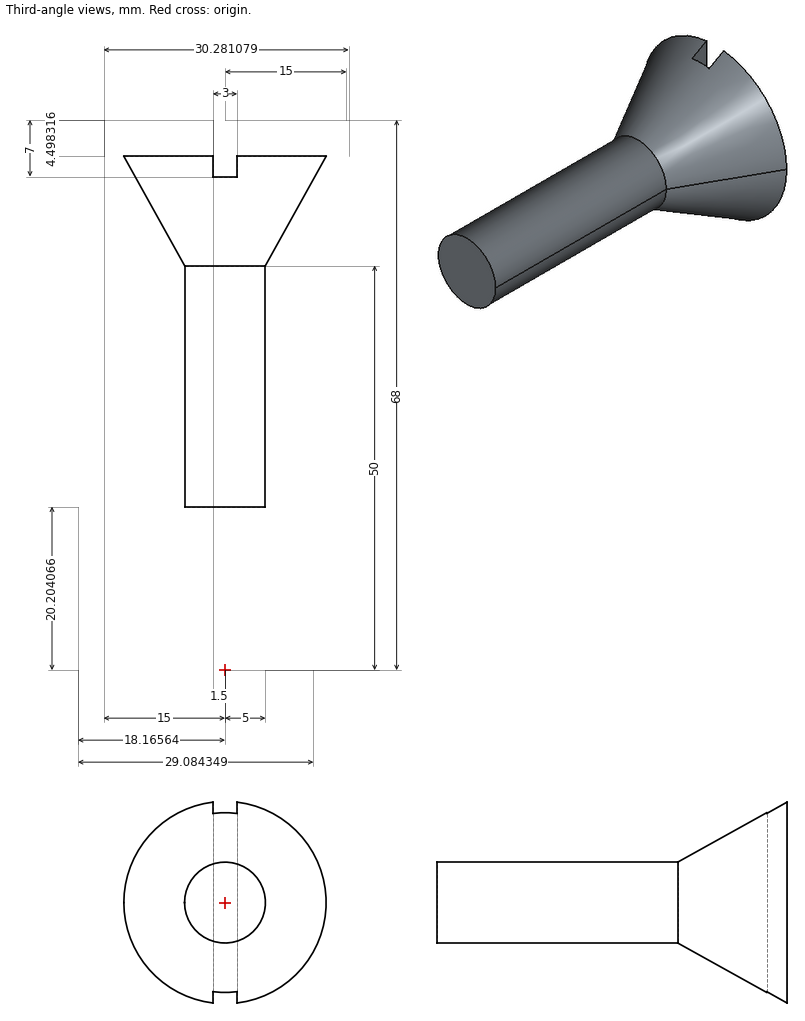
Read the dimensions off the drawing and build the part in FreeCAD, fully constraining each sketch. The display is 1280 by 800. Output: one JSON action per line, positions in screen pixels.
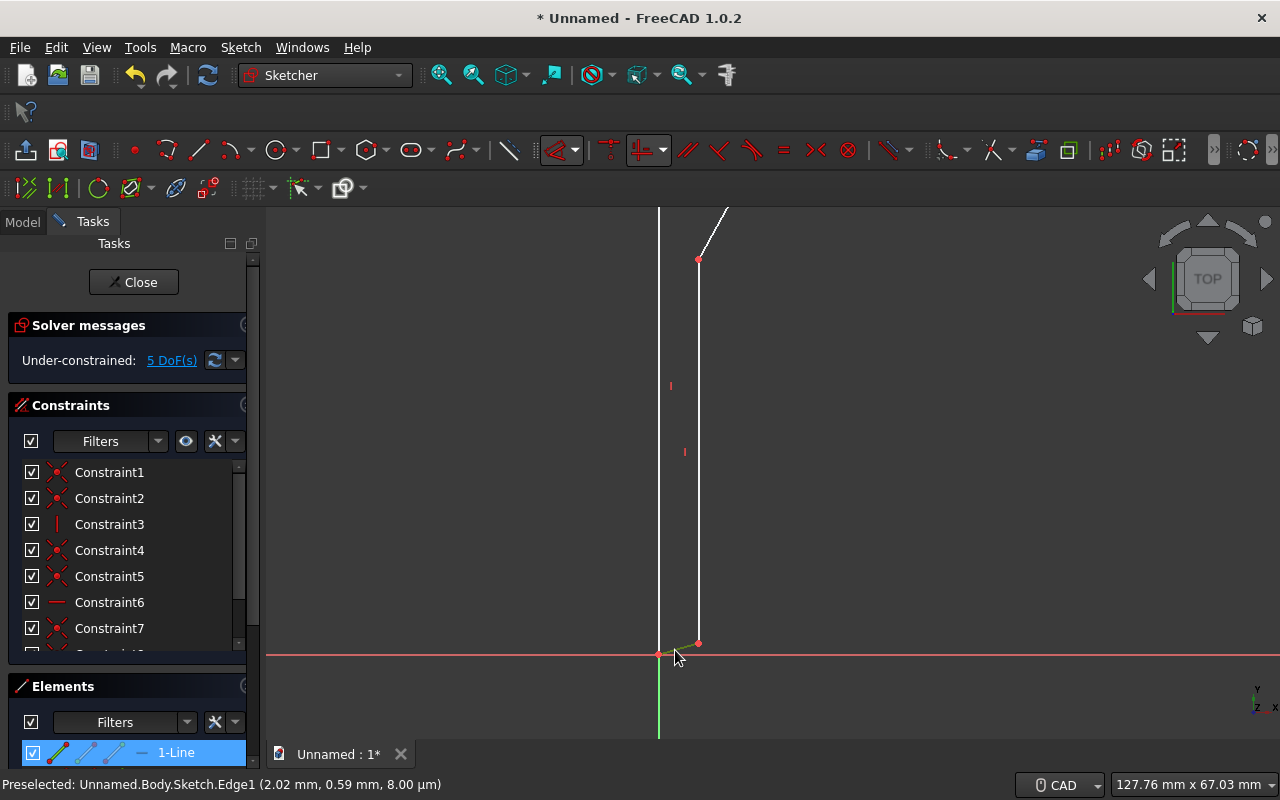
{"action": "left_click", "coordinate": [666, 150]}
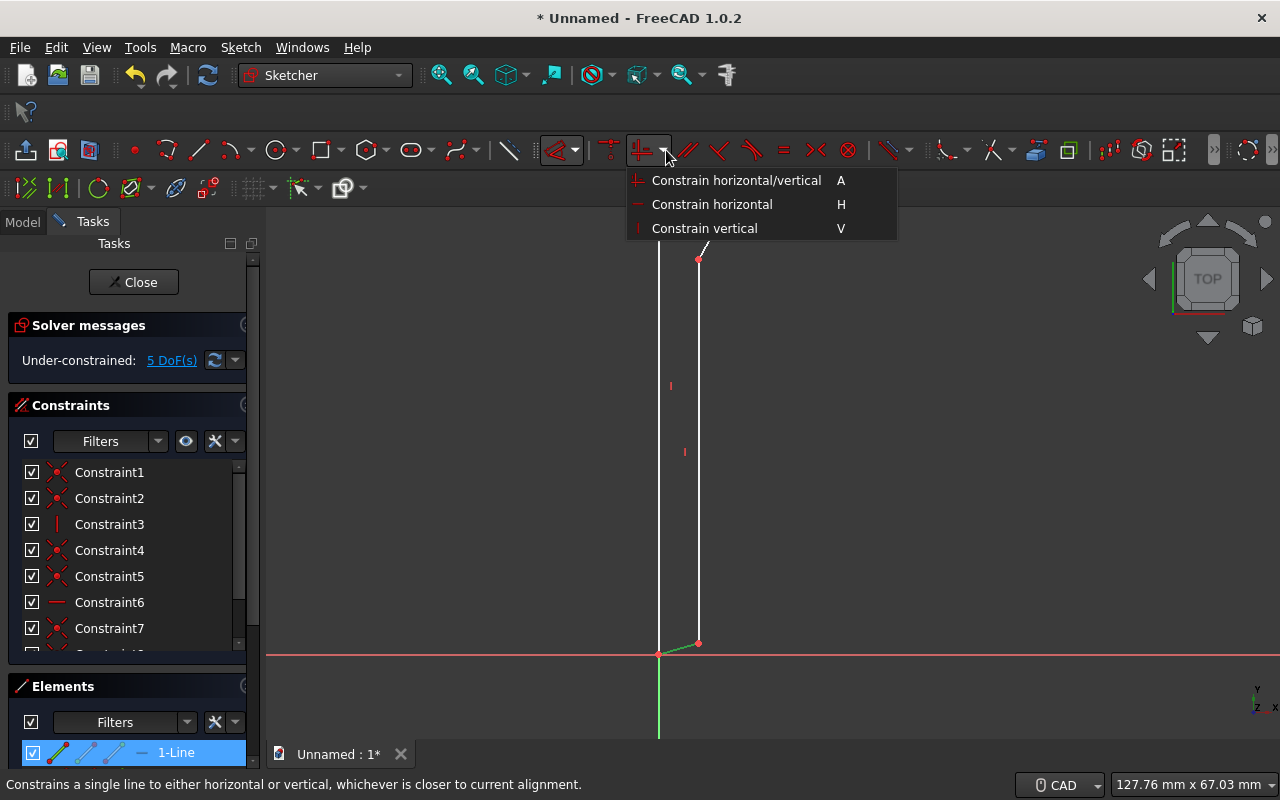
{"action": "left_click", "coordinate": [762, 204]}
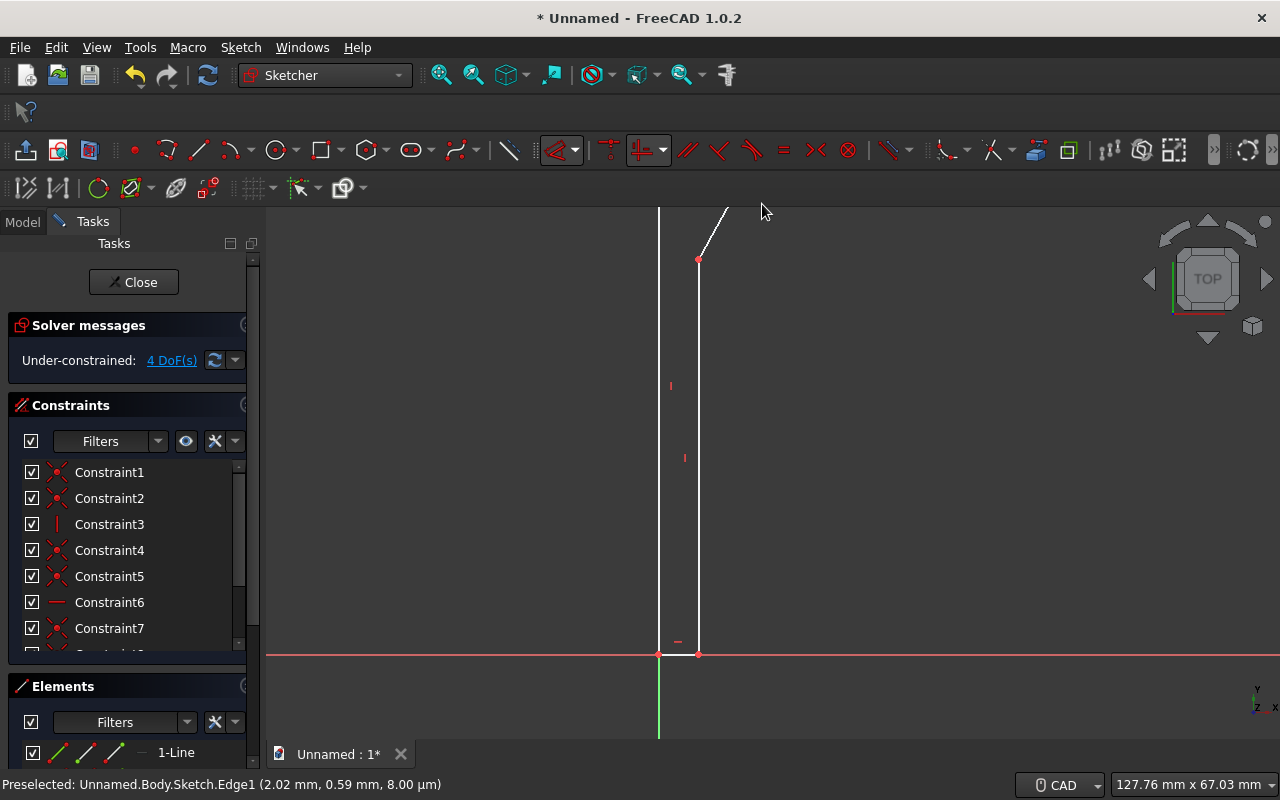
{"action": "left_click", "coordinate": [556, 150]}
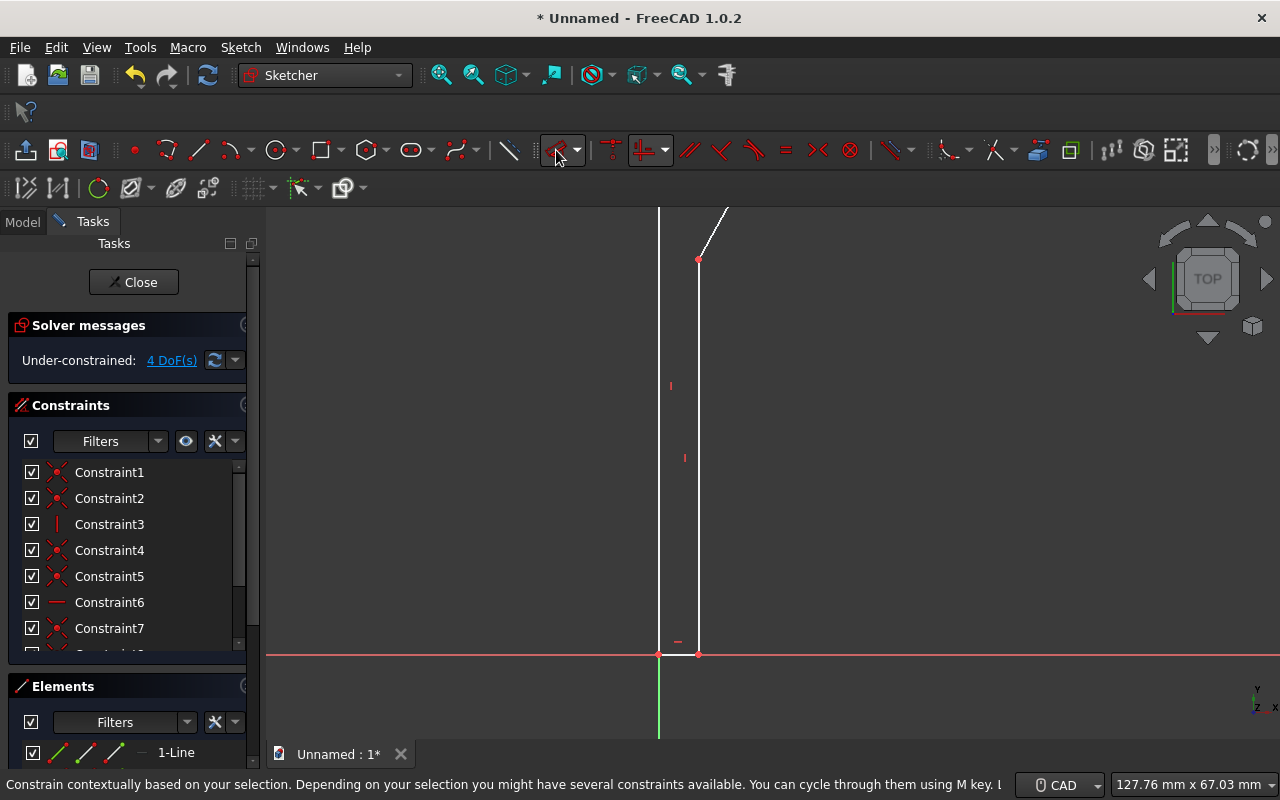
{"action": "left_click", "coordinate": [671, 655]}
{"action": "left_click", "coordinate": [679, 689]}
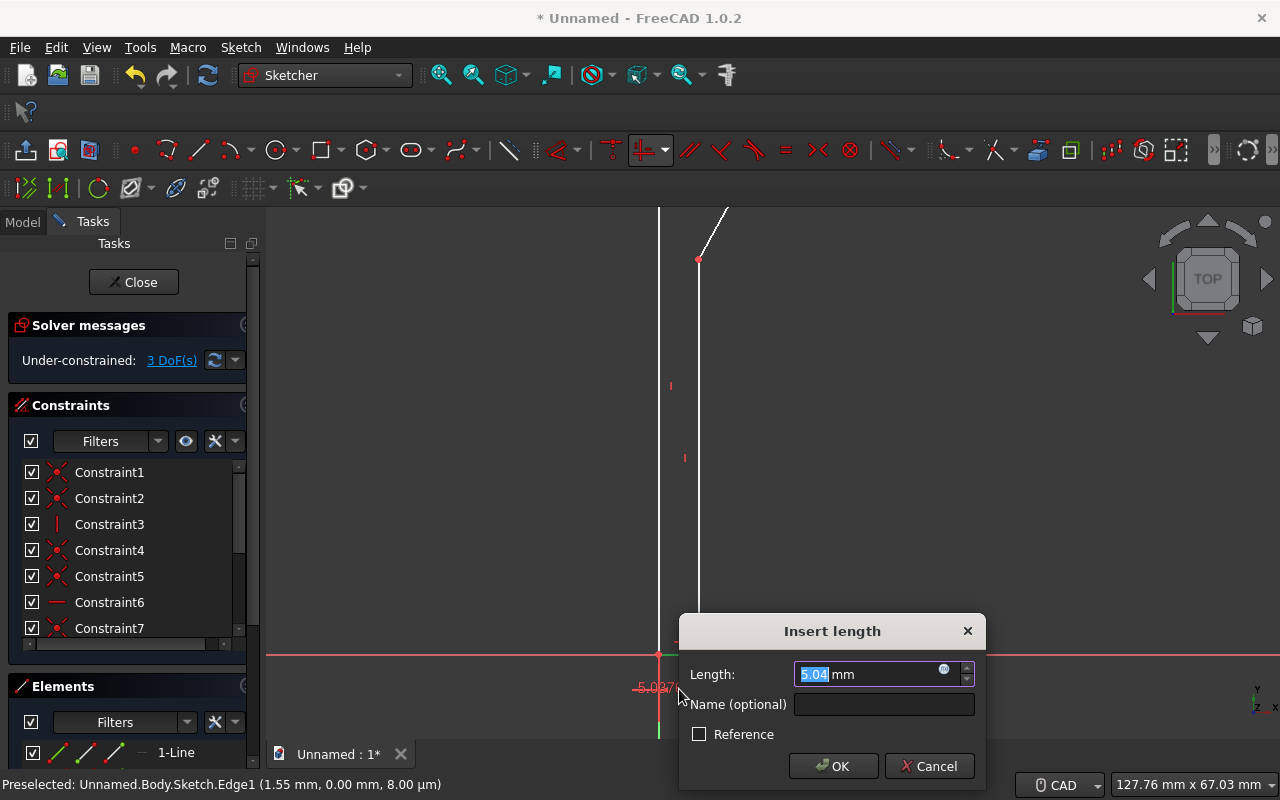
{"action": "type", "text": "5"}
{"action": "key", "text": "Return"}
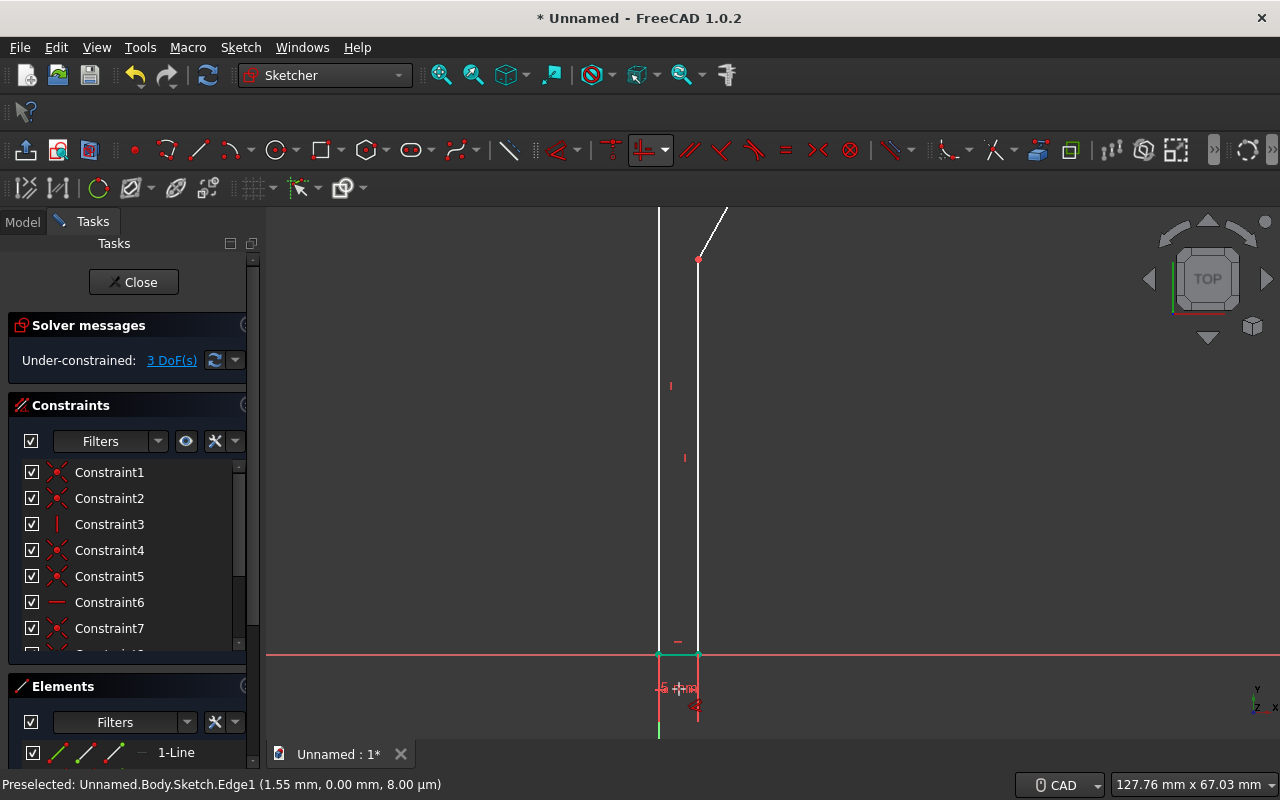
{"action": "left_click", "coordinate": [698, 536]}
{"action": "left_click", "coordinate": [732, 457]}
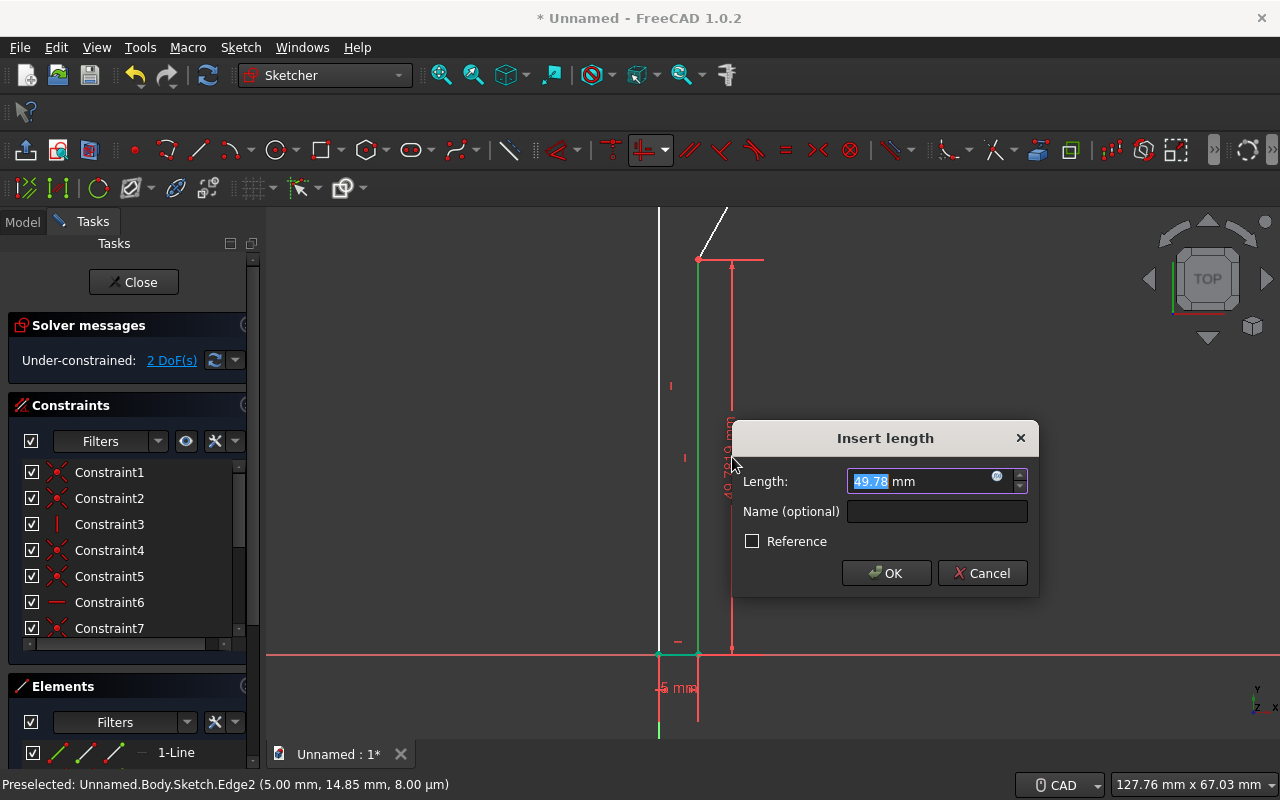
{"action": "type", "text": "50"}
{"action": "key", "text": "Return"}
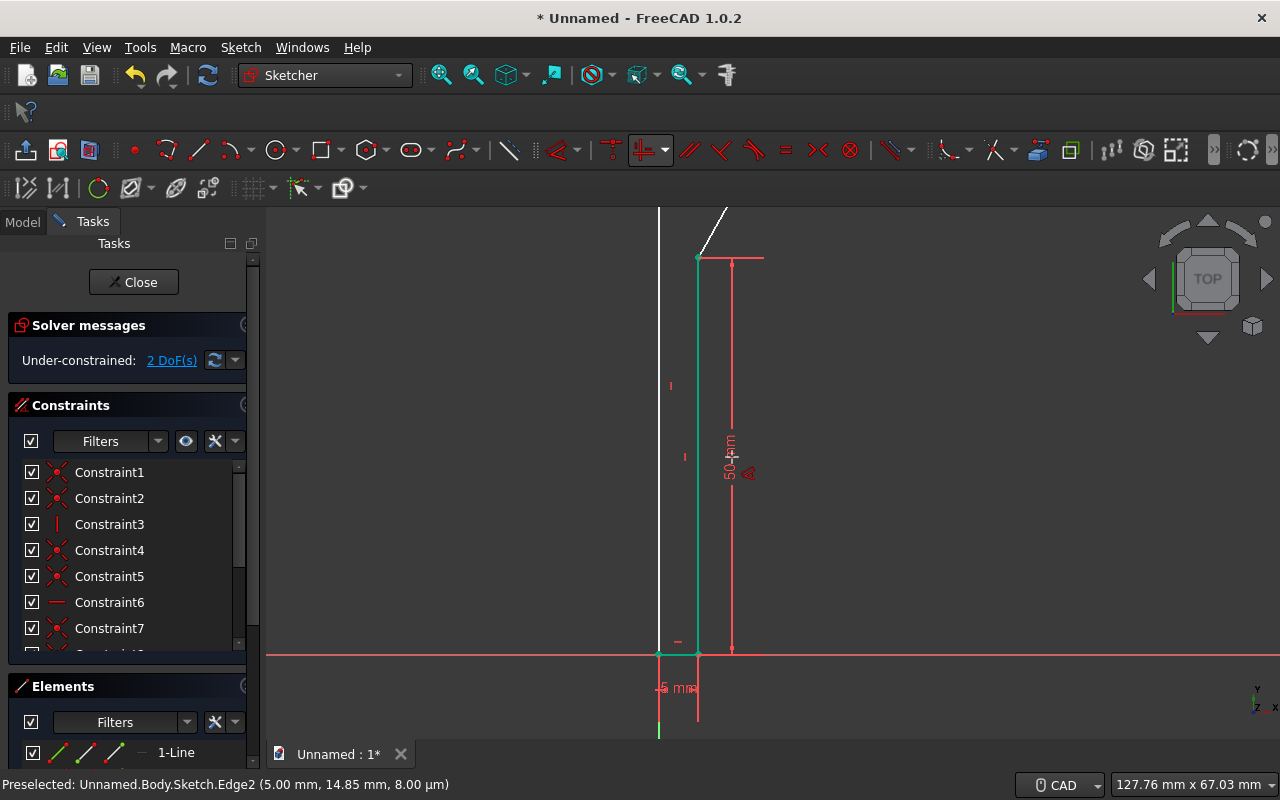
{"action": "scroll", "coordinate": [677, 652], "scroll_direction": "down", "scroll_amount": 2}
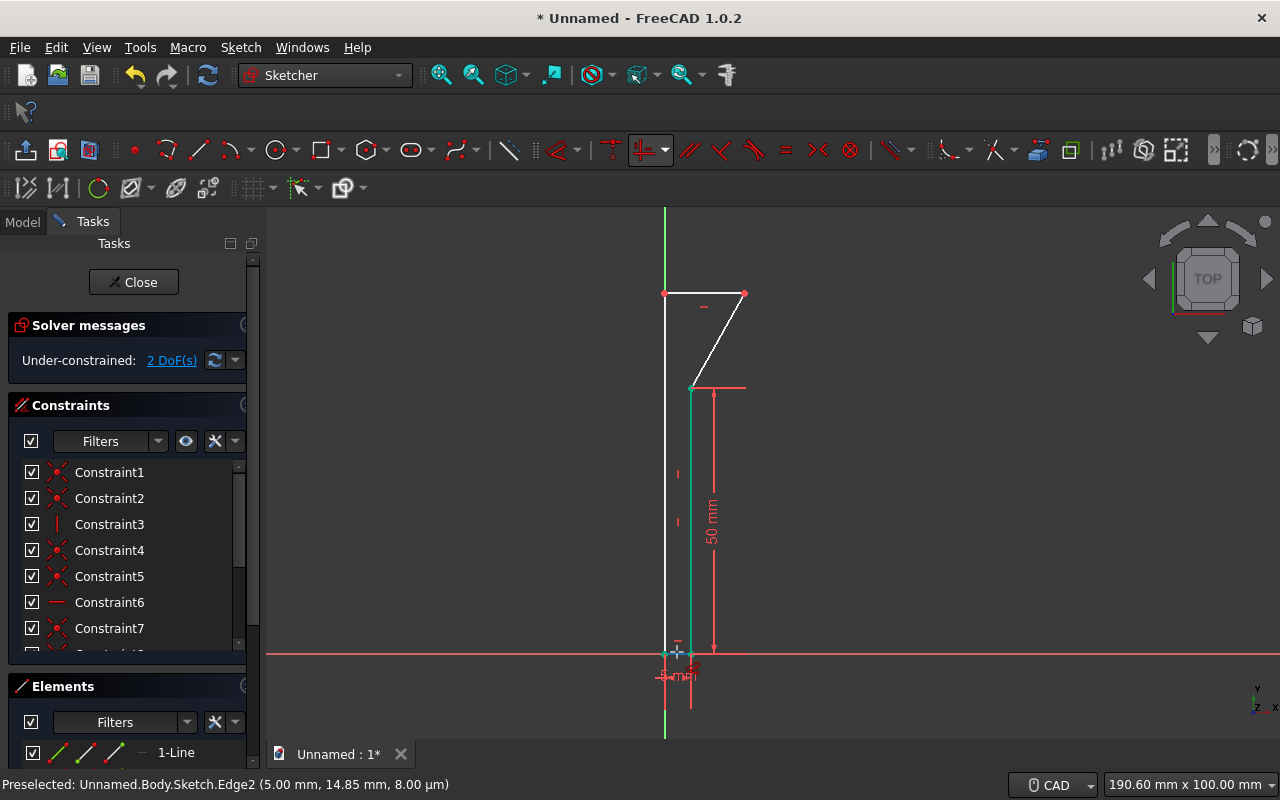
{"action": "left_click", "coordinate": [721, 293]}
{"action": "left_click", "coordinate": [705, 259]}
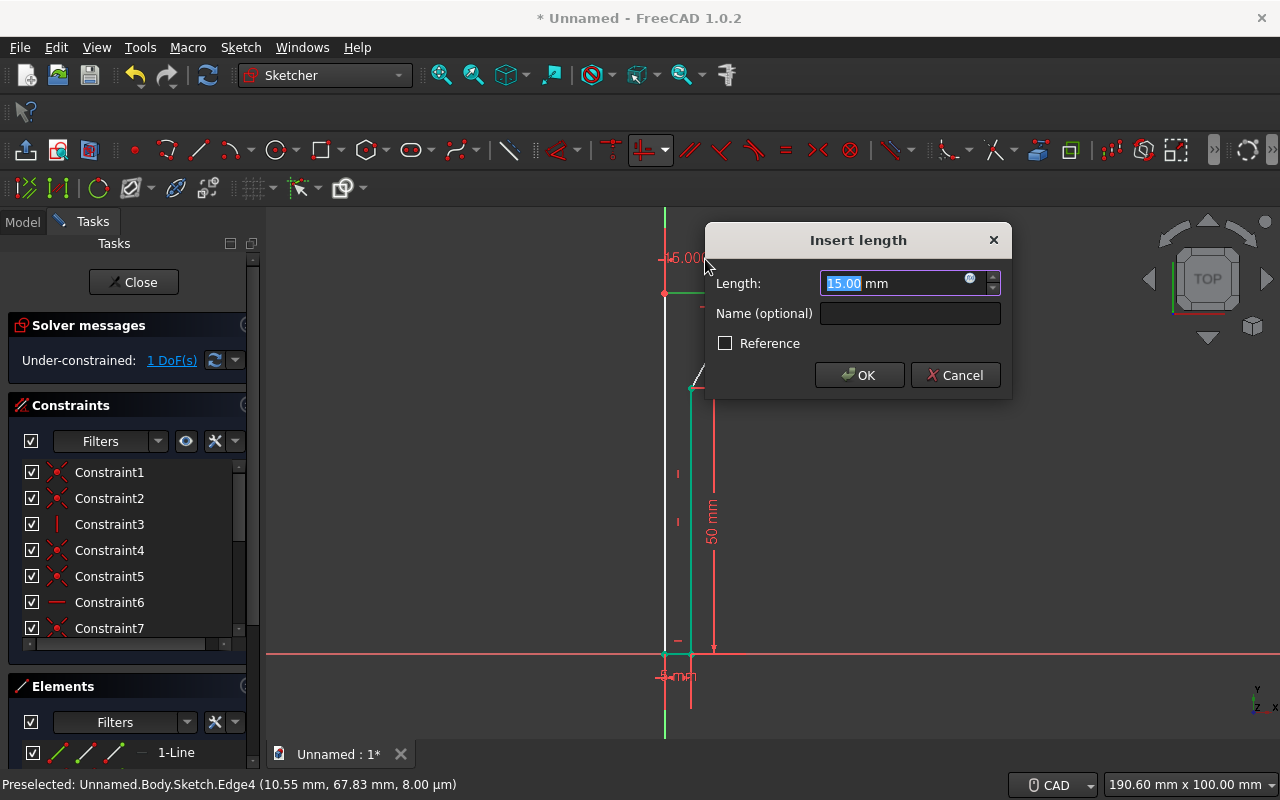
{"action": "type", "text": "15"}
{"action": "key", "text": "Return"}